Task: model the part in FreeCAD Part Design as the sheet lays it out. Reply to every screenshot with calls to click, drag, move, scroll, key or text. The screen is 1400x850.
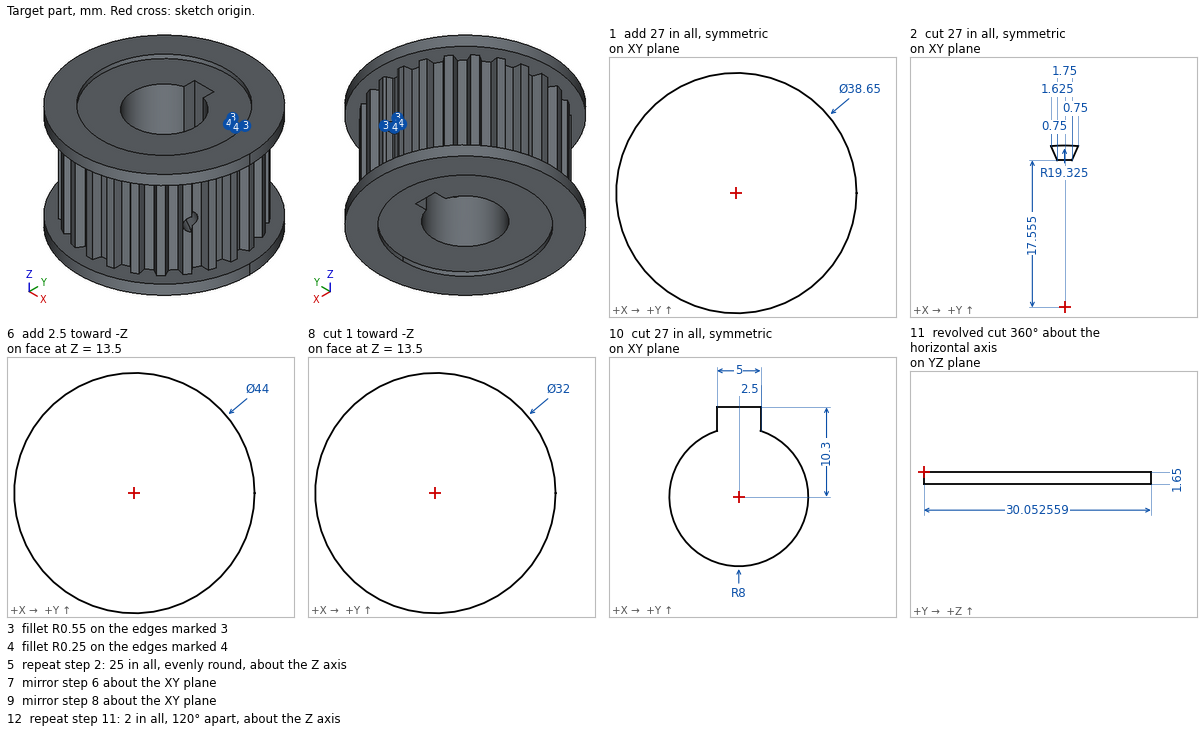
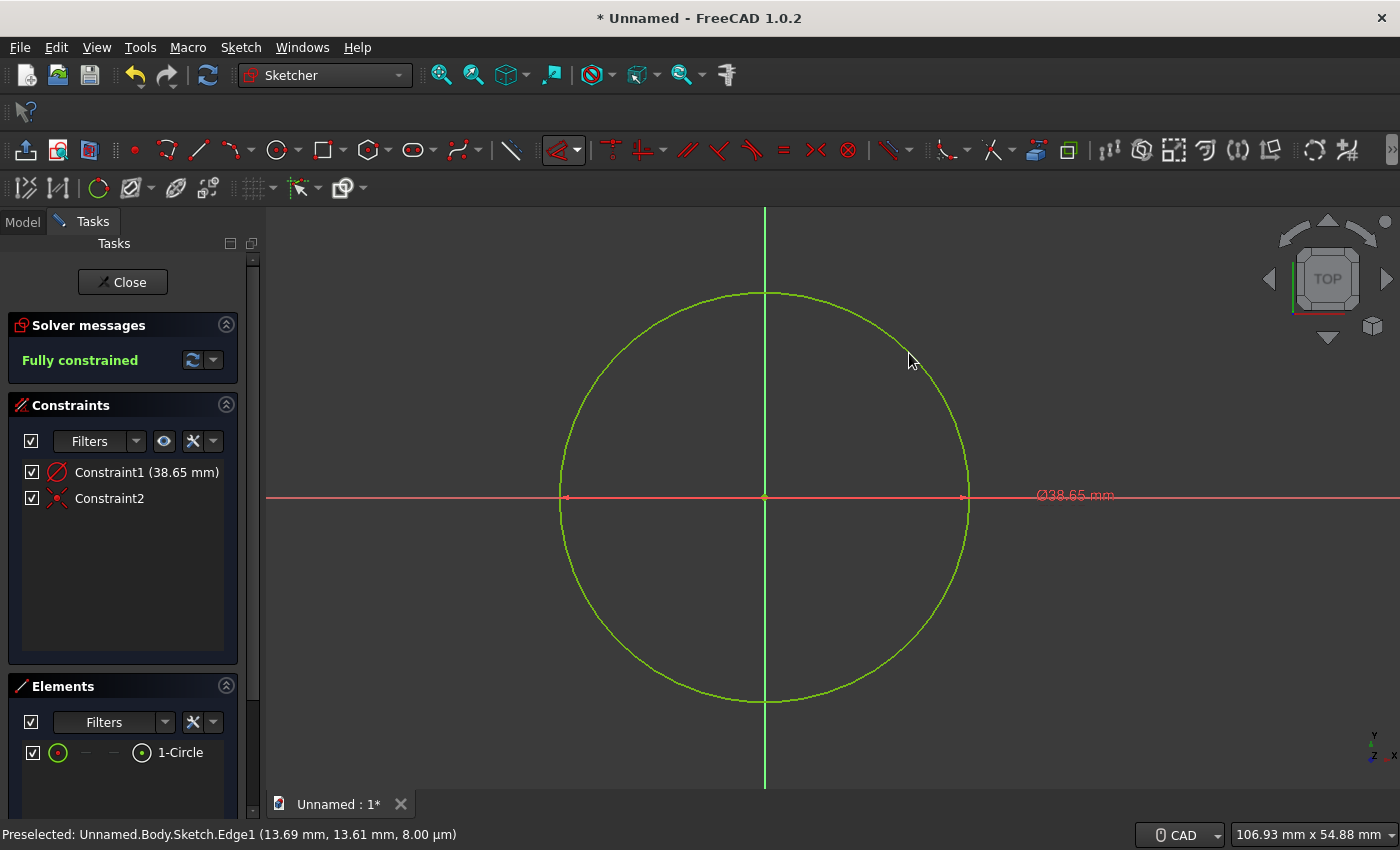
click(123, 282)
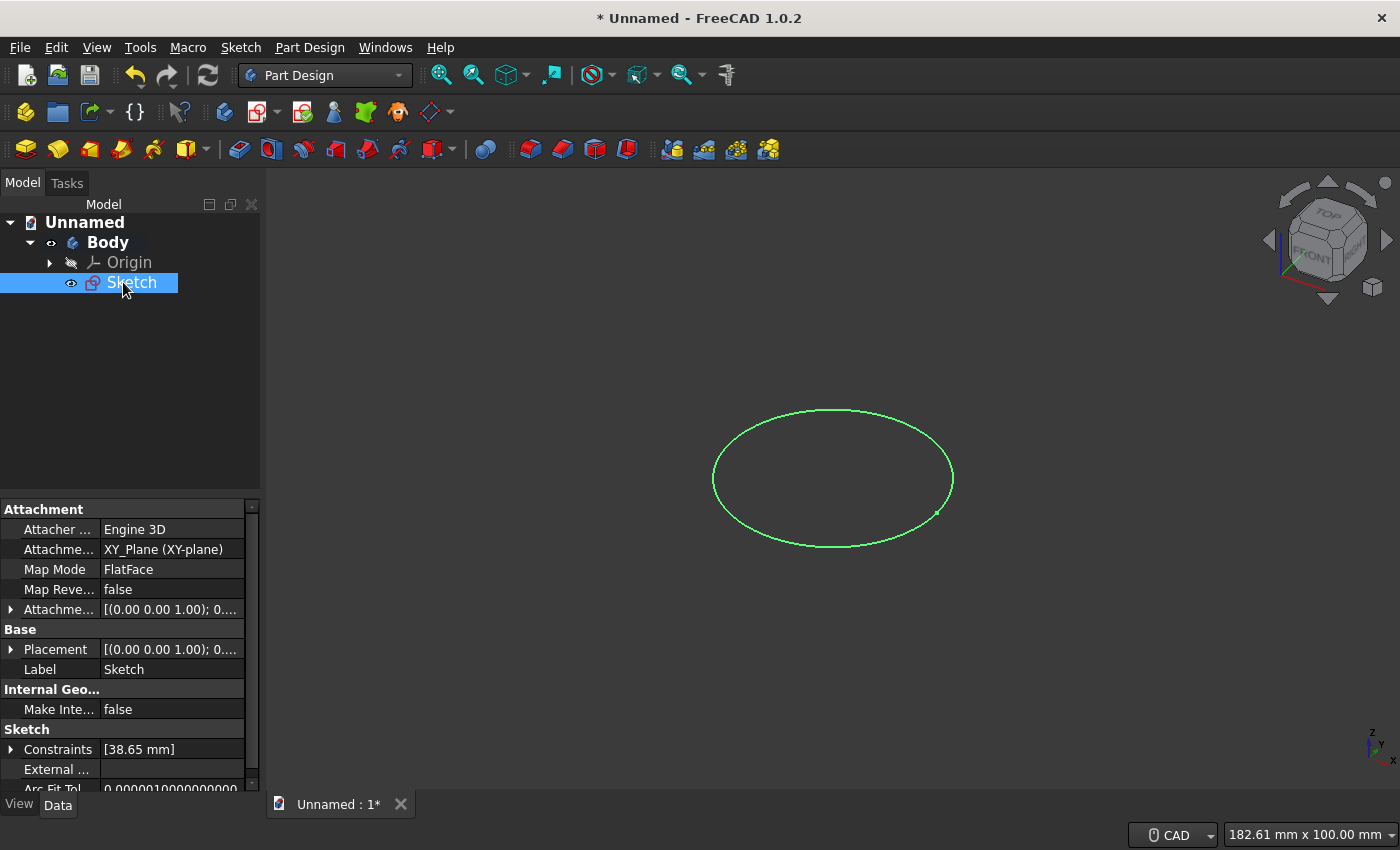
click(26, 150)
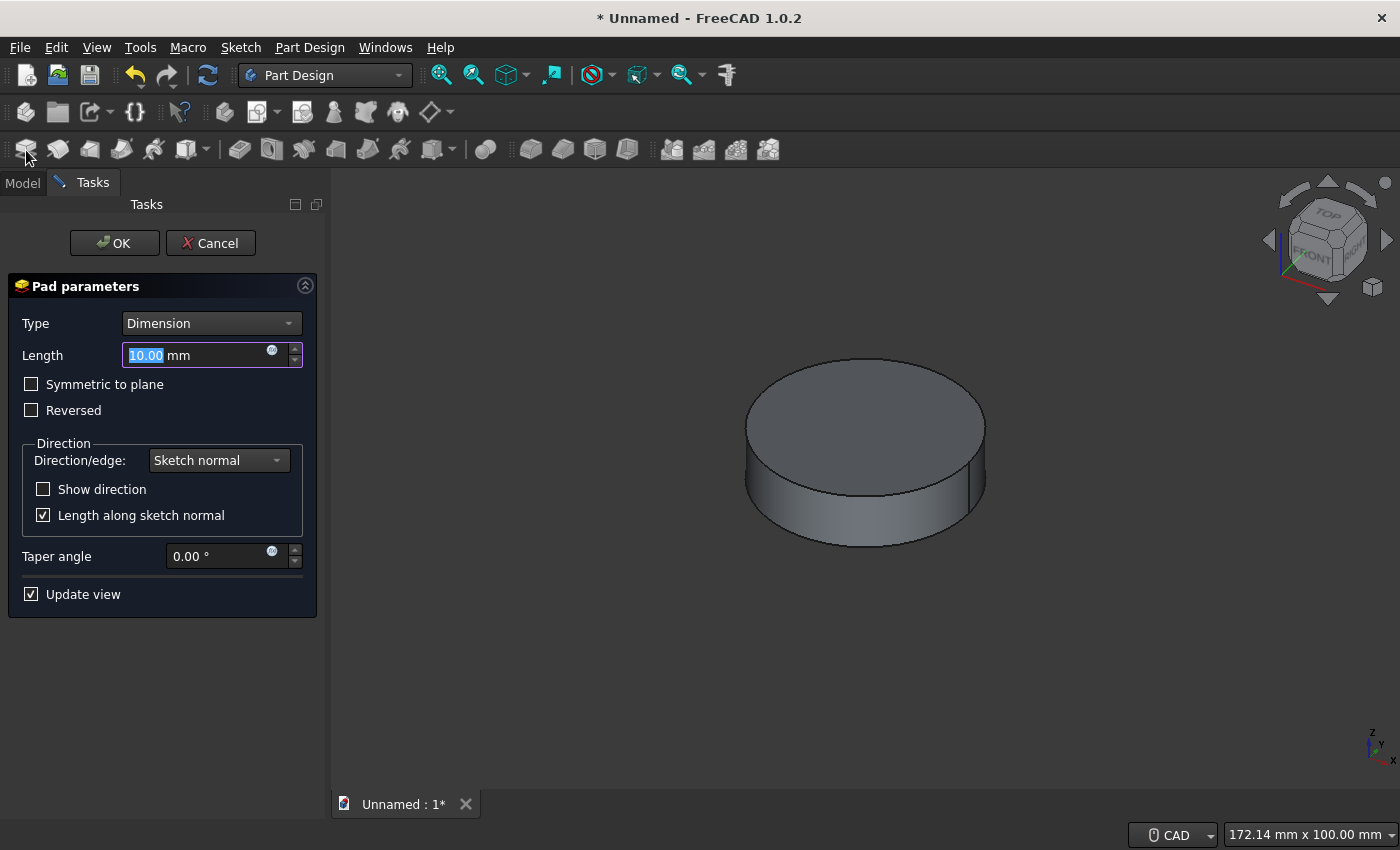
text(27)
key(Tab)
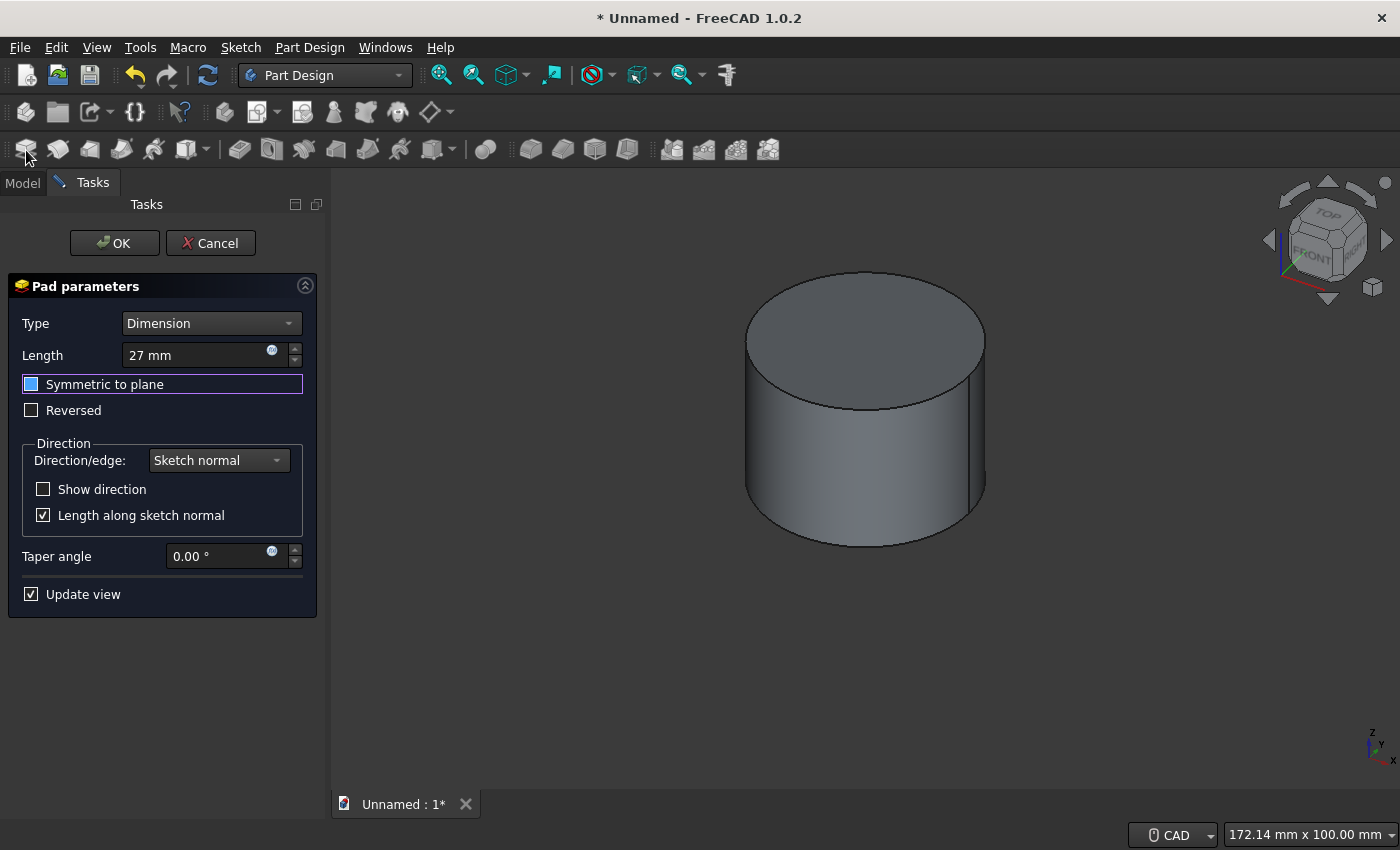
click(30, 384)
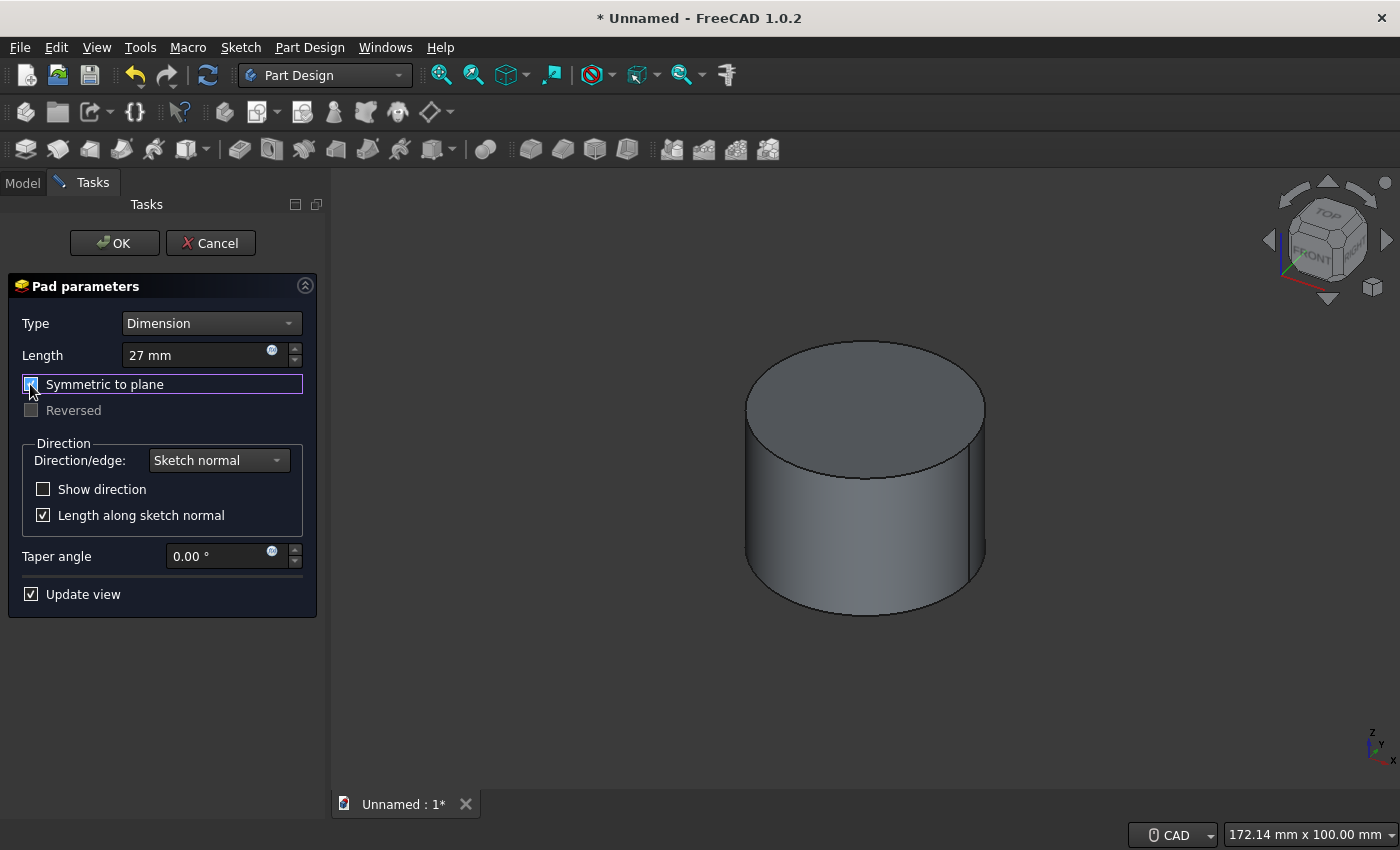
click(115, 243)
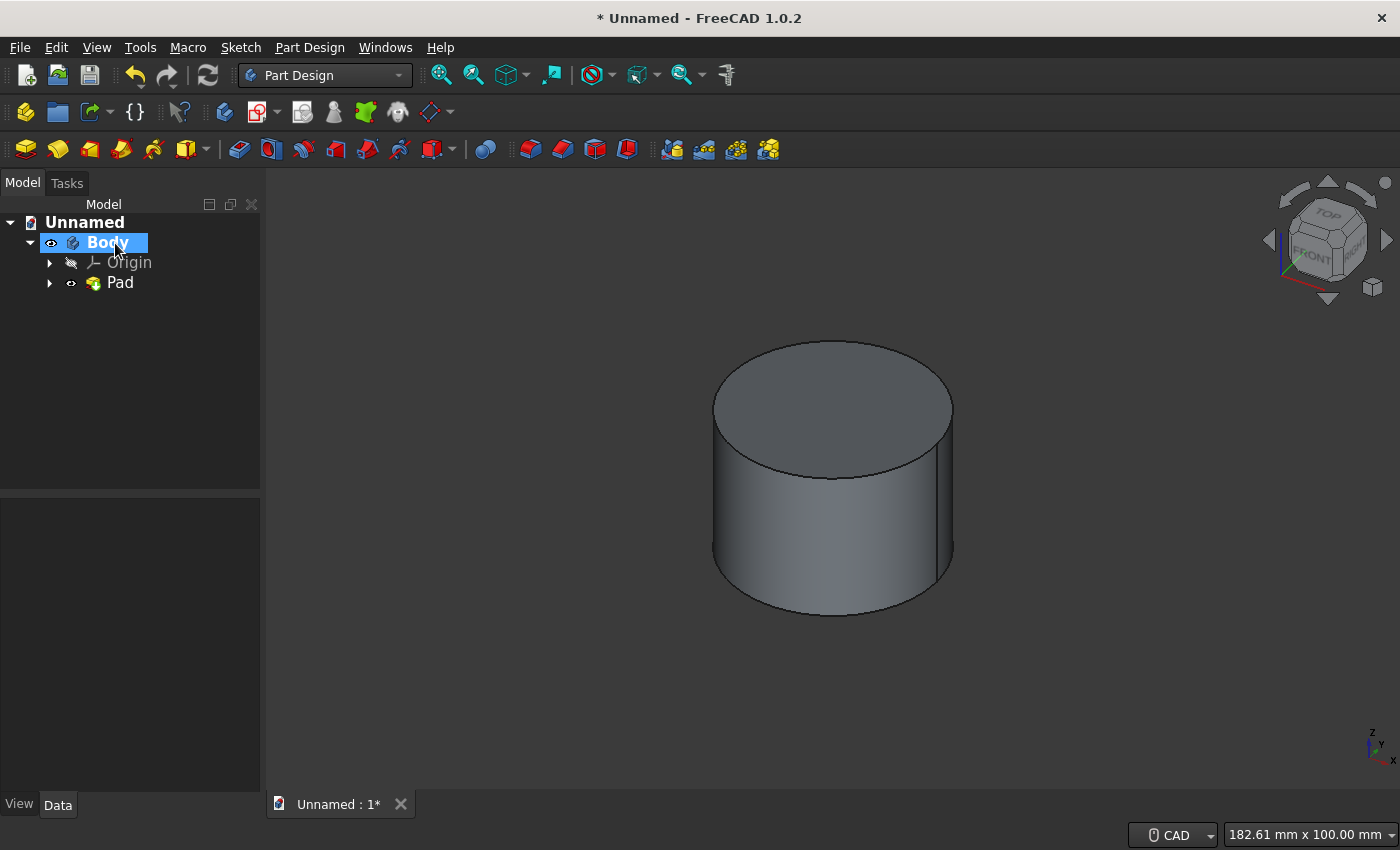
click(258, 112)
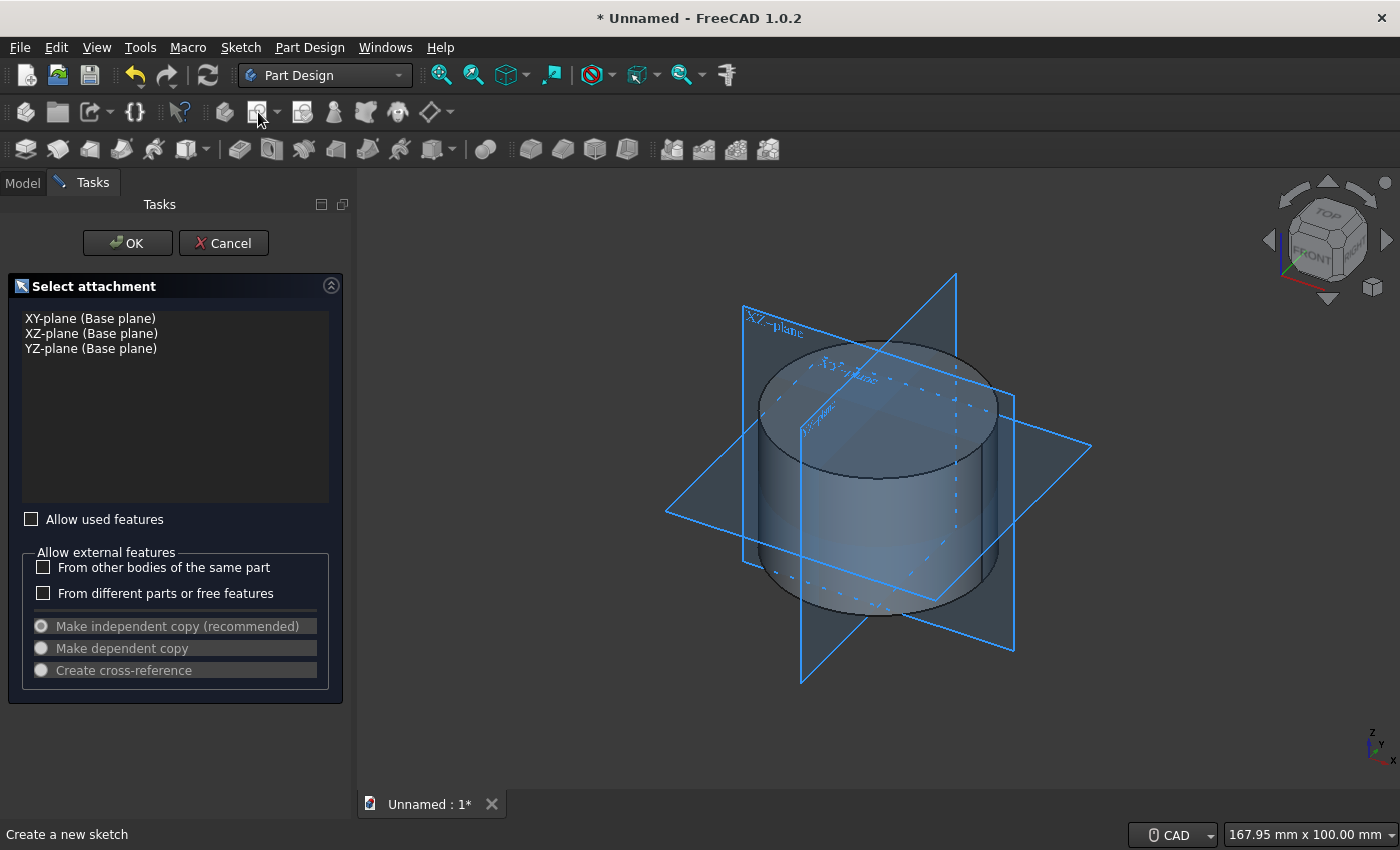
click(82, 318)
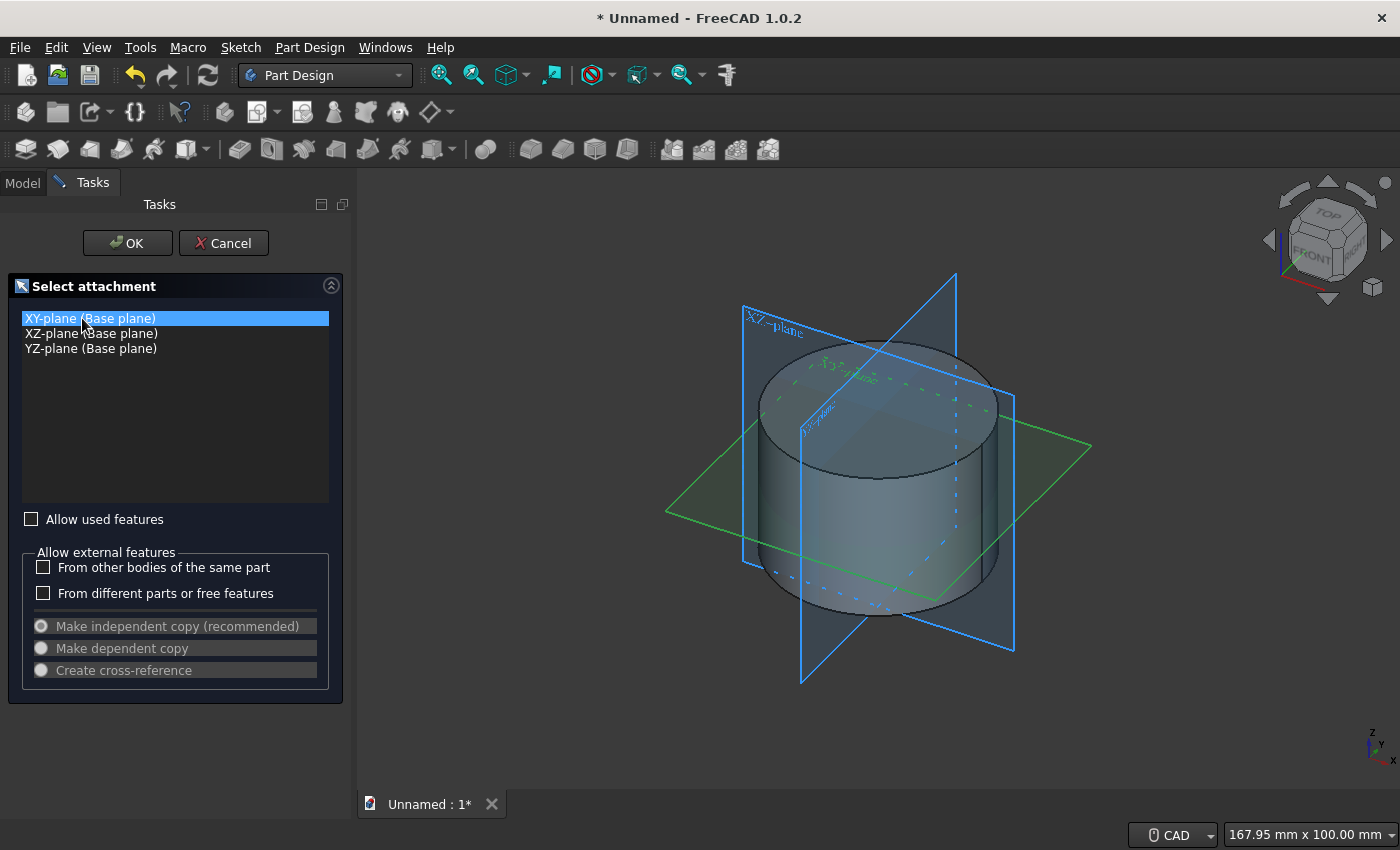
click(128, 243)